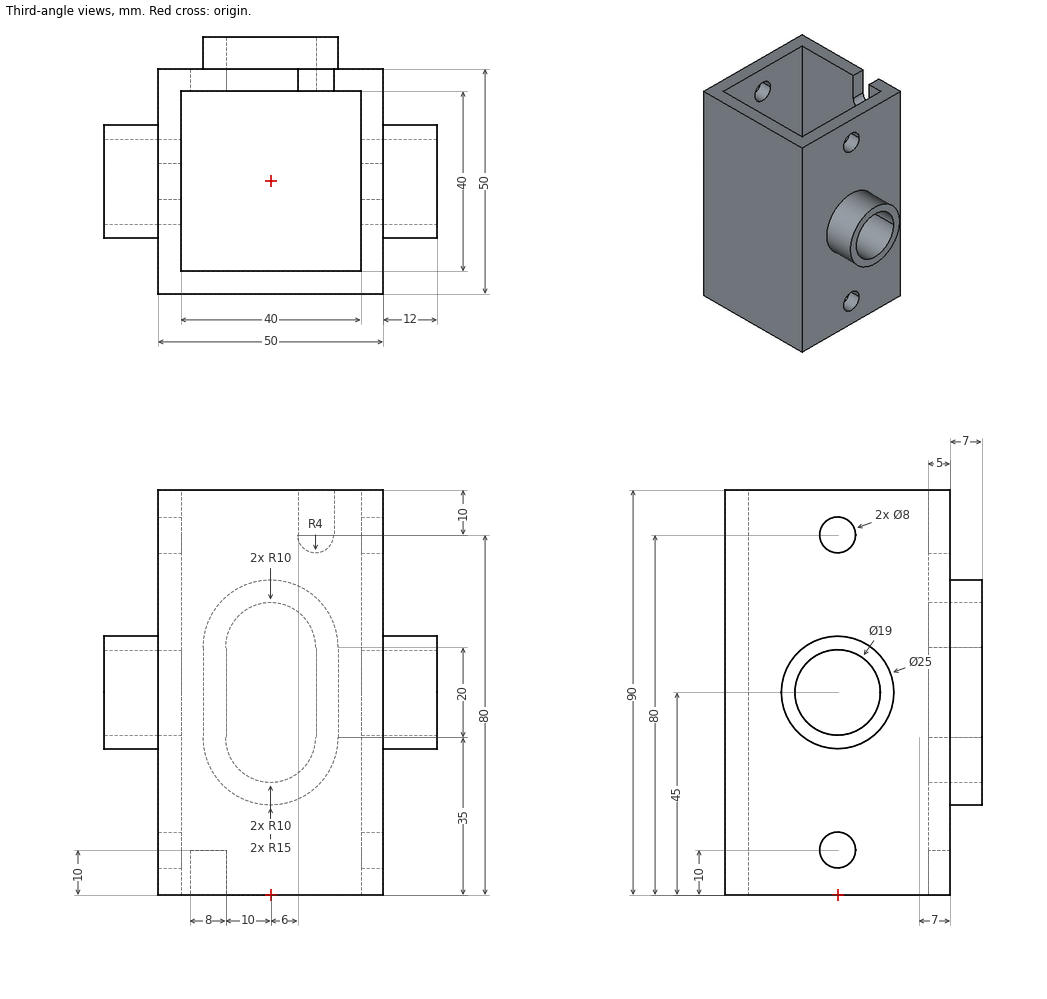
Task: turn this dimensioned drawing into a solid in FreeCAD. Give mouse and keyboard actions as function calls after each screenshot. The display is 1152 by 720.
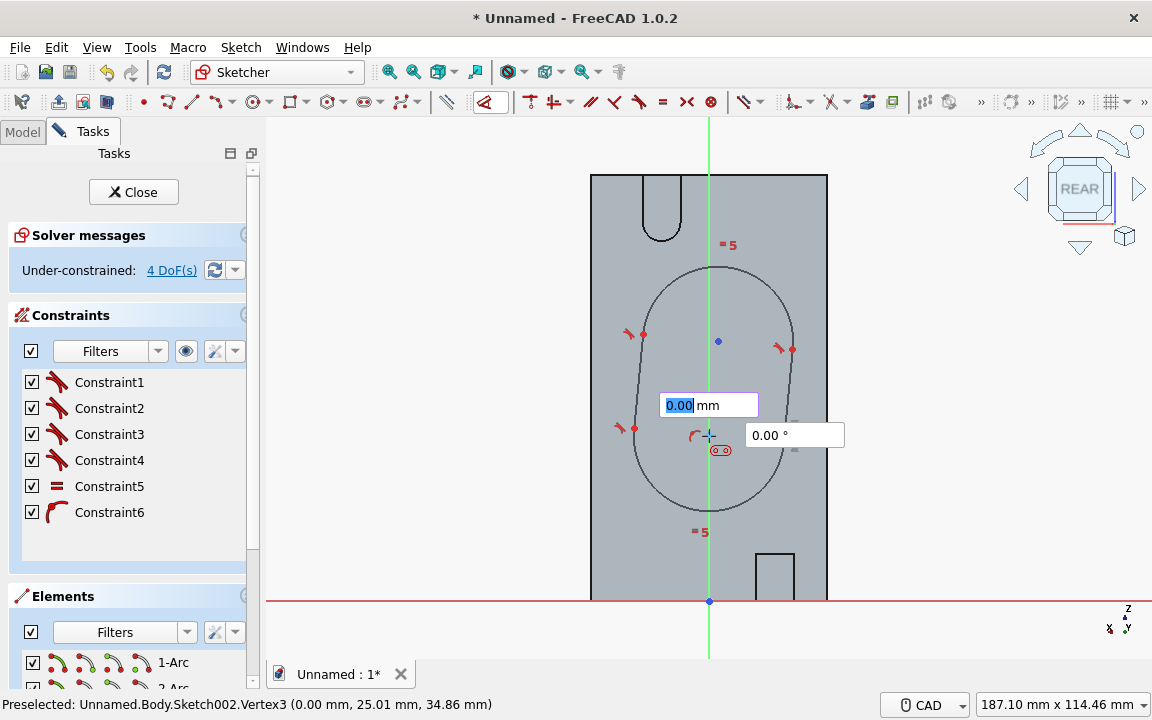
click(718, 342)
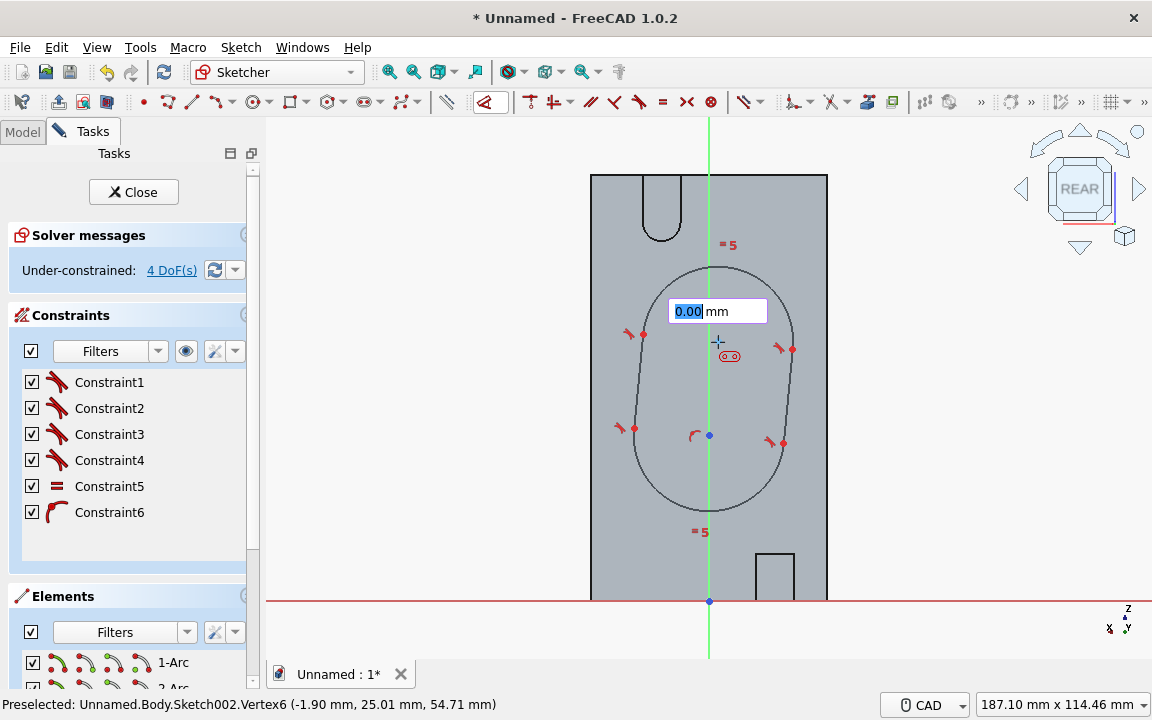
click(662, 388)
key(Escape)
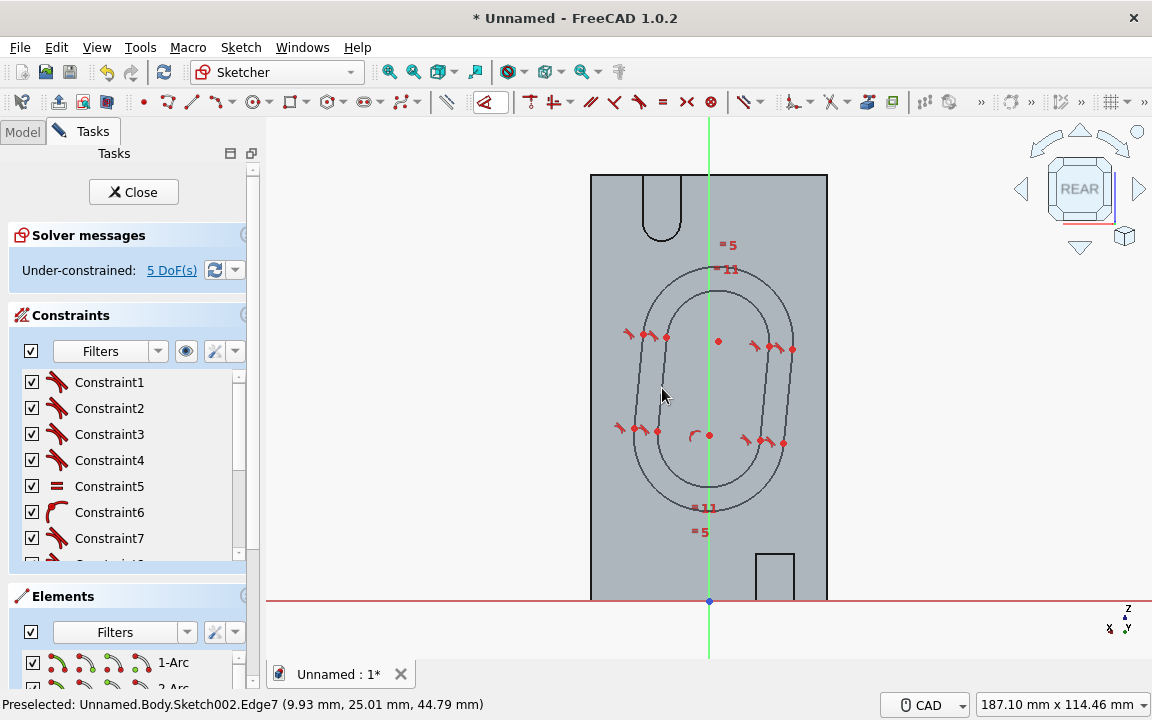
click(637, 401)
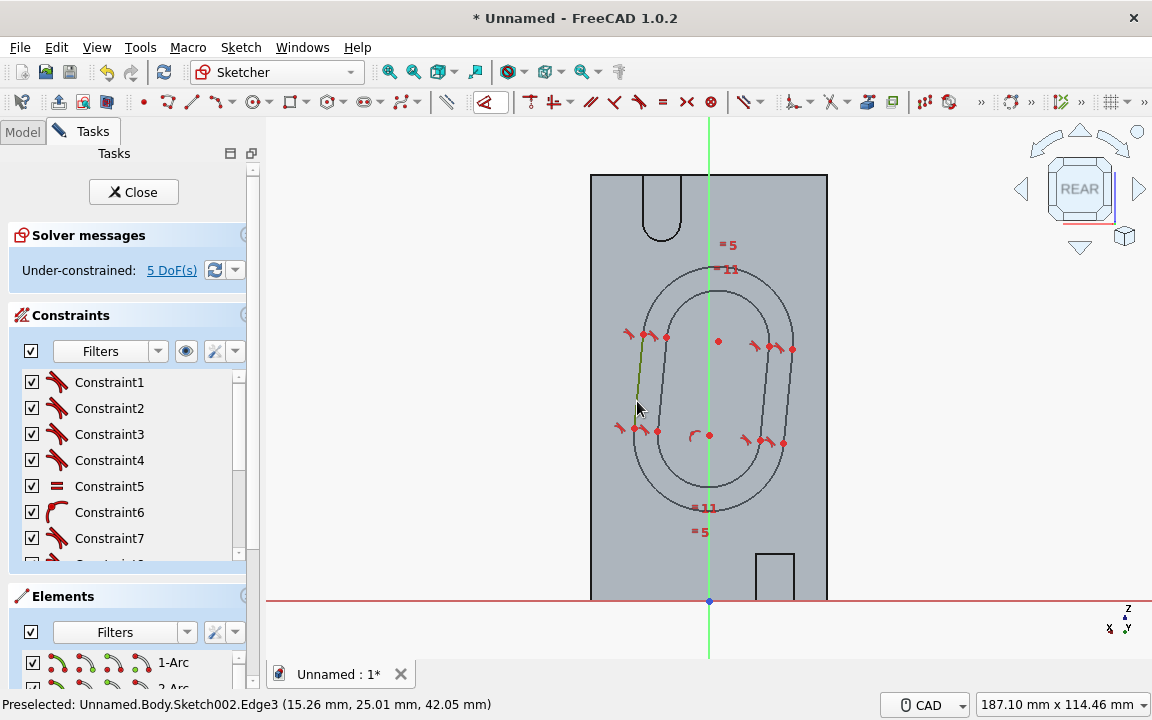
key(v)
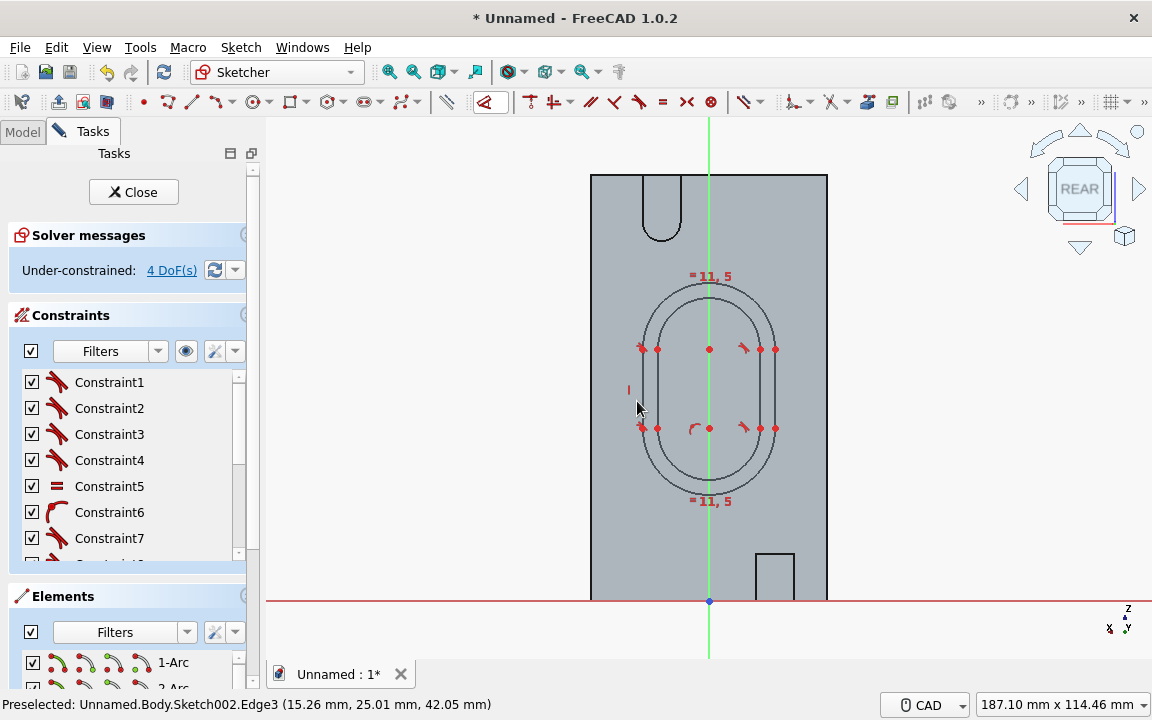
click(484, 102)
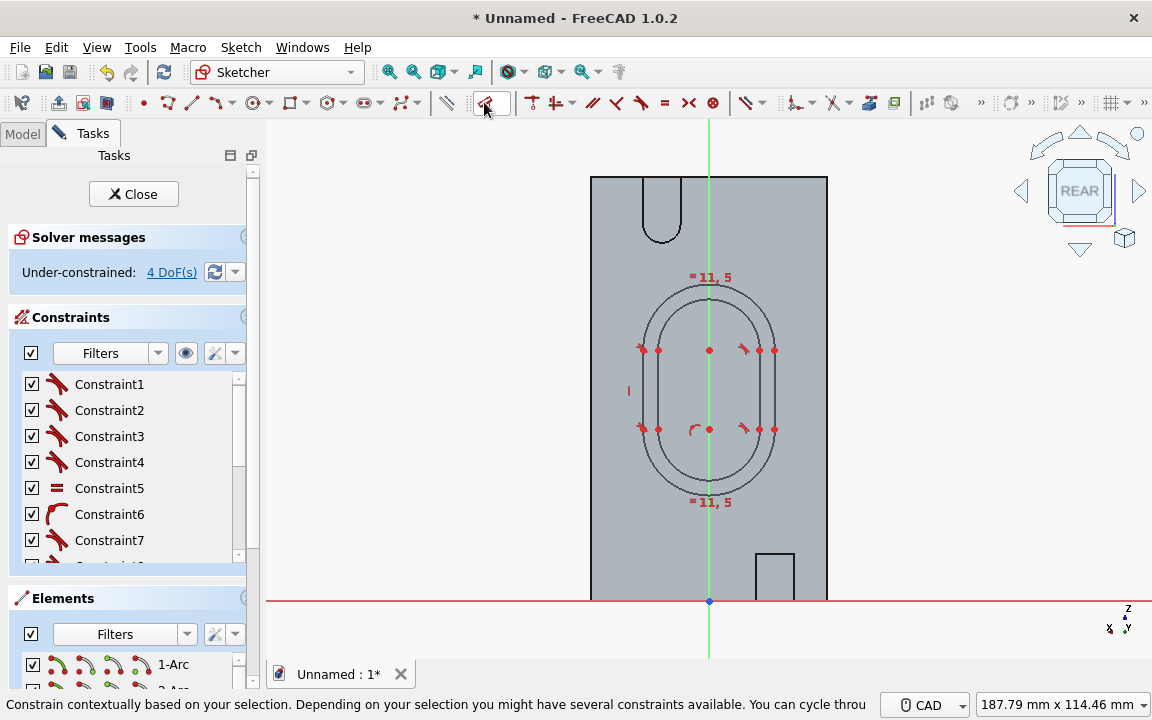
click(670, 483)
click(651, 509)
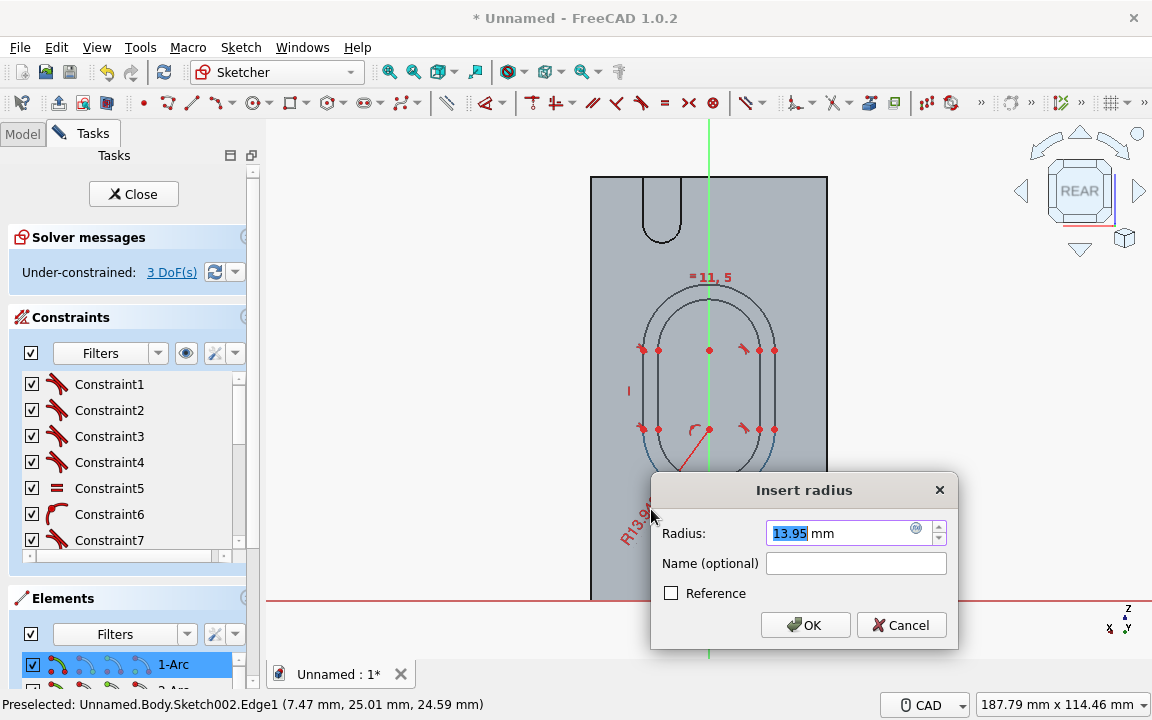
text(15)
key(Return)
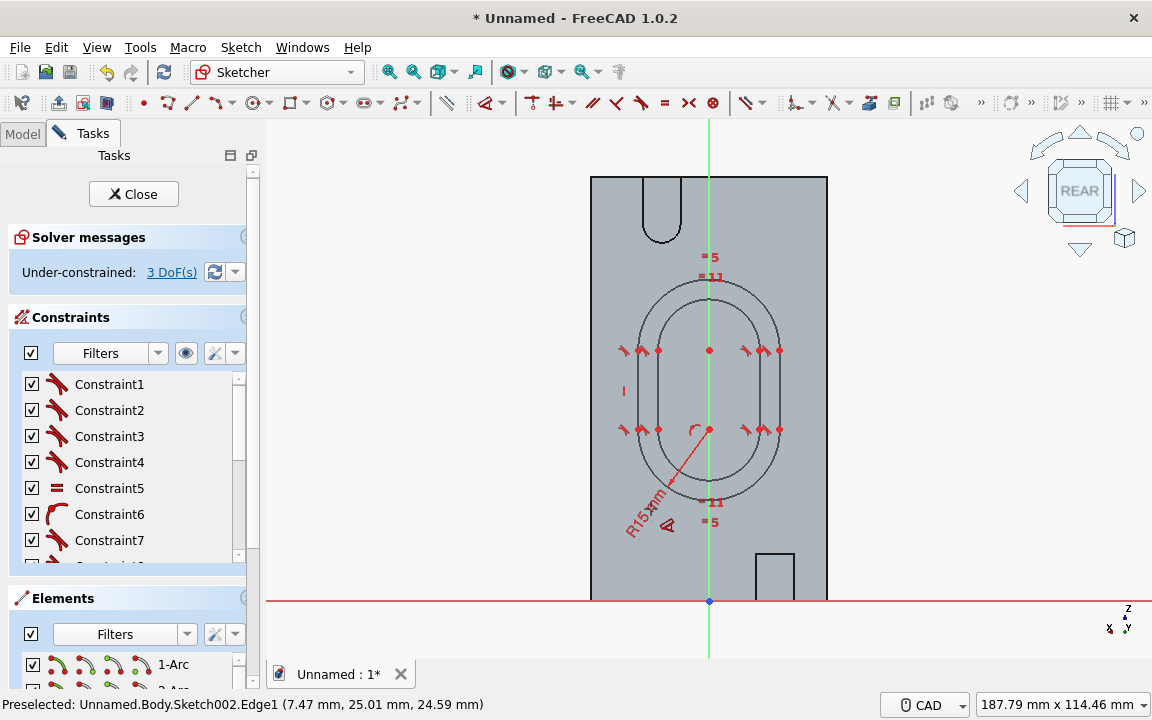
click(679, 471)
click(613, 475)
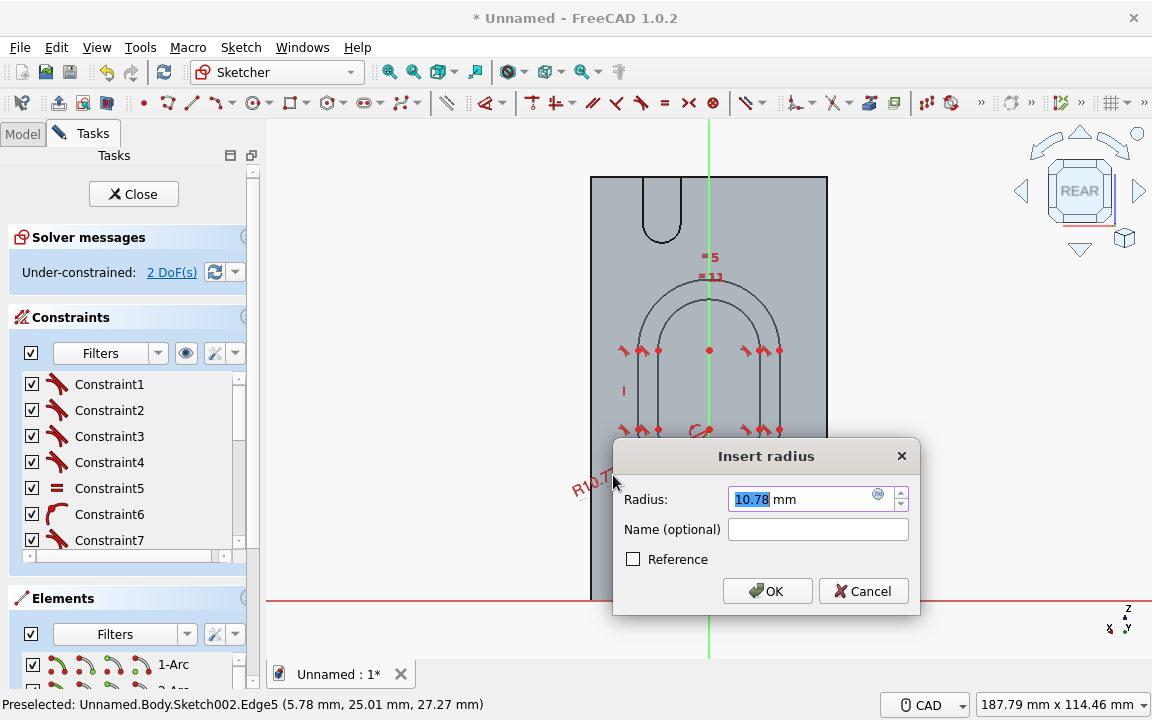
text(10)
key(Return)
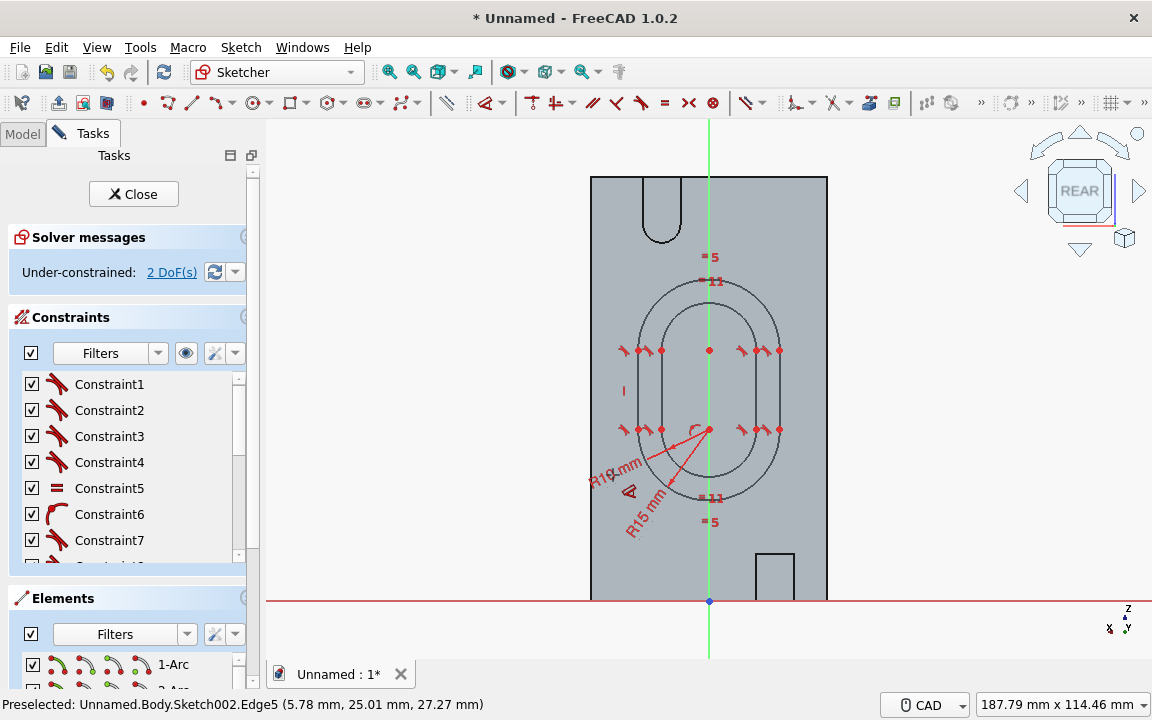
click(638, 406)
click(604, 390)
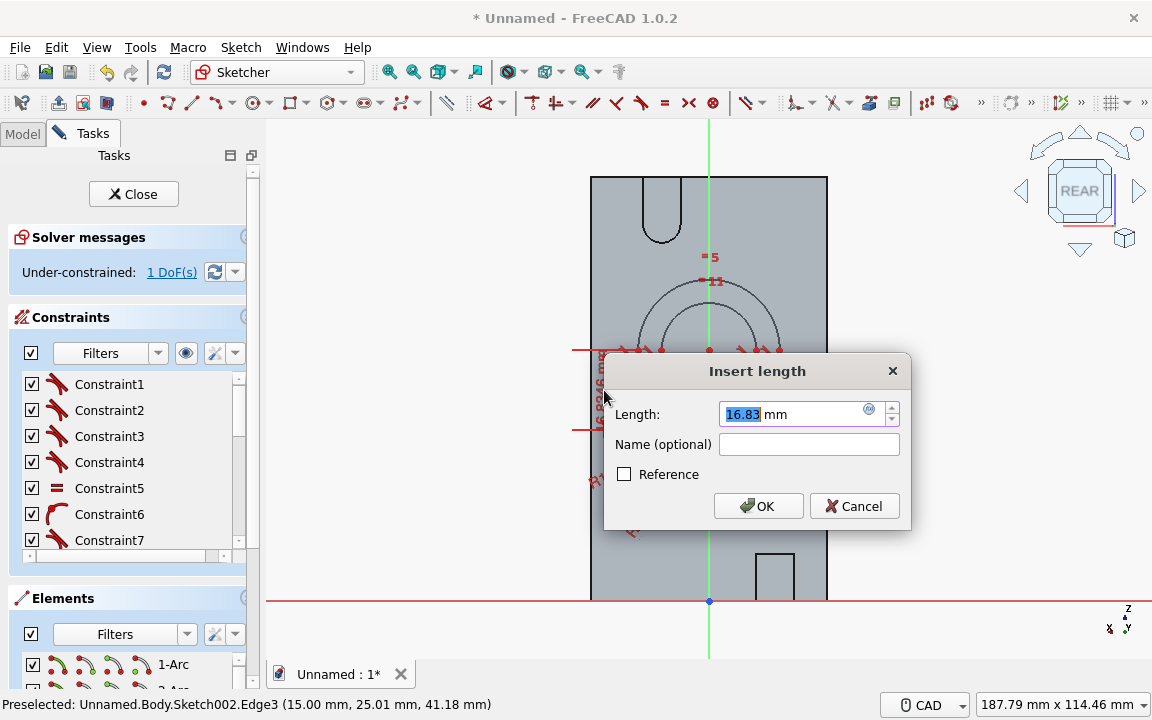
text(20)
key(Return)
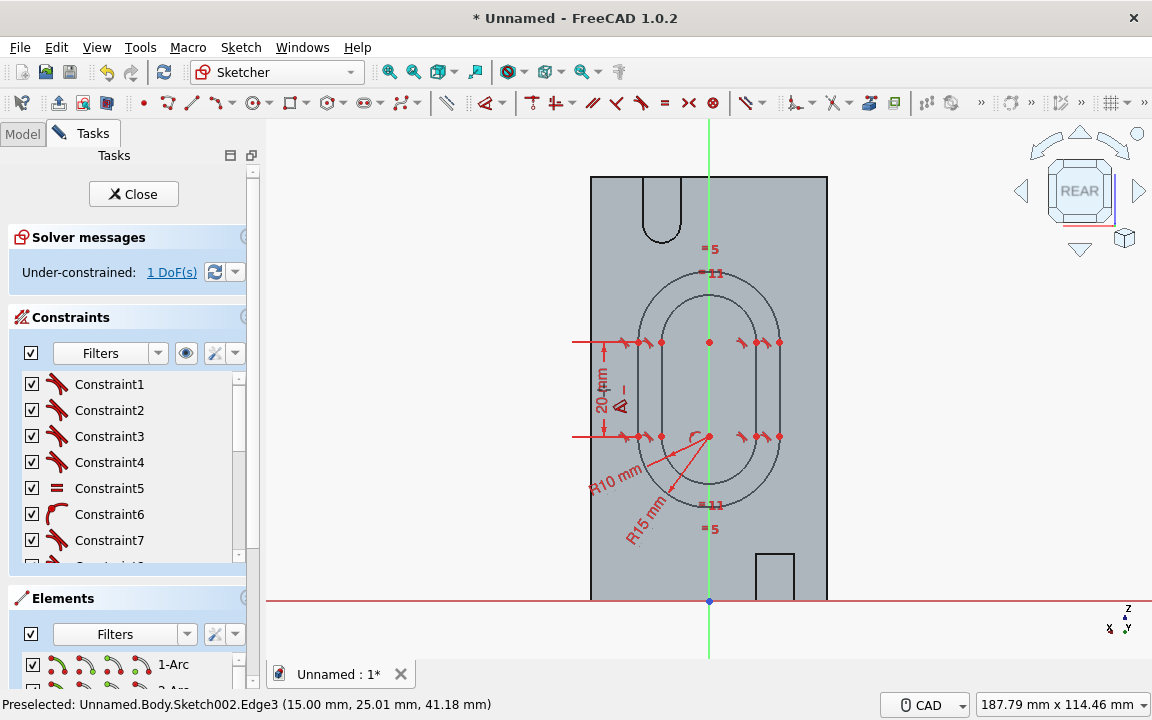
click(638, 437)
click(604, 557)